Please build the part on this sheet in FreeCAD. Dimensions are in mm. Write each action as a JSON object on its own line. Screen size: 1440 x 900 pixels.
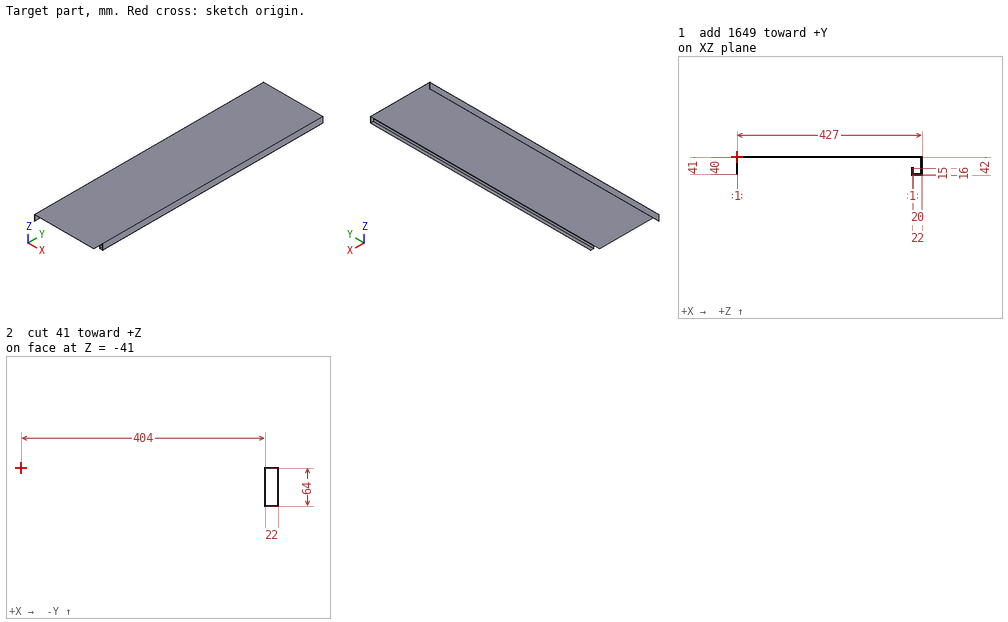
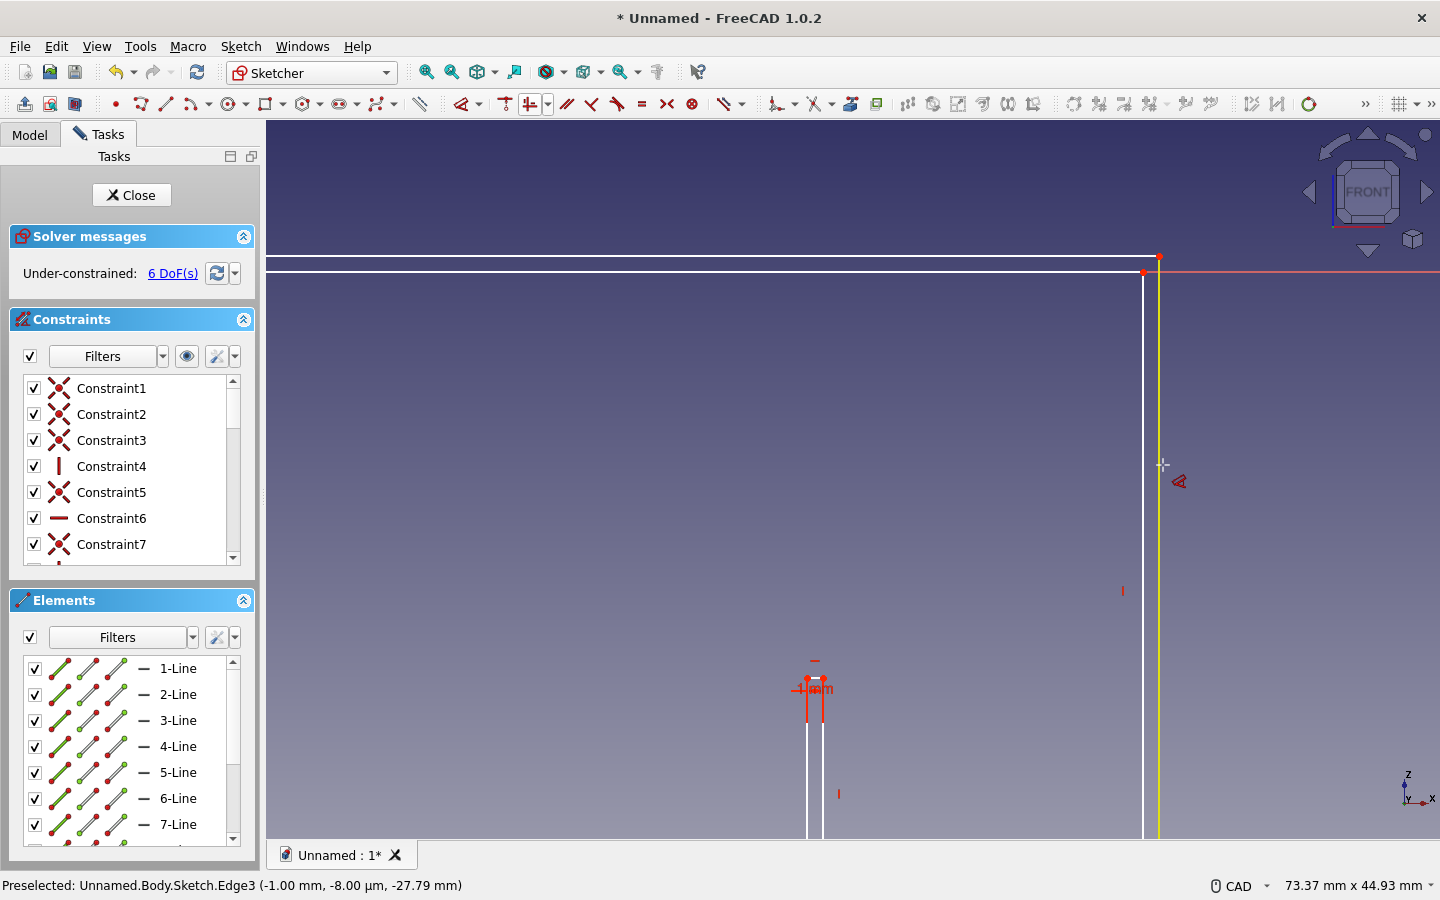
{"action": "left_click", "coordinate": [1159, 461]}
{"action": "left_click", "coordinate": [1193, 534]}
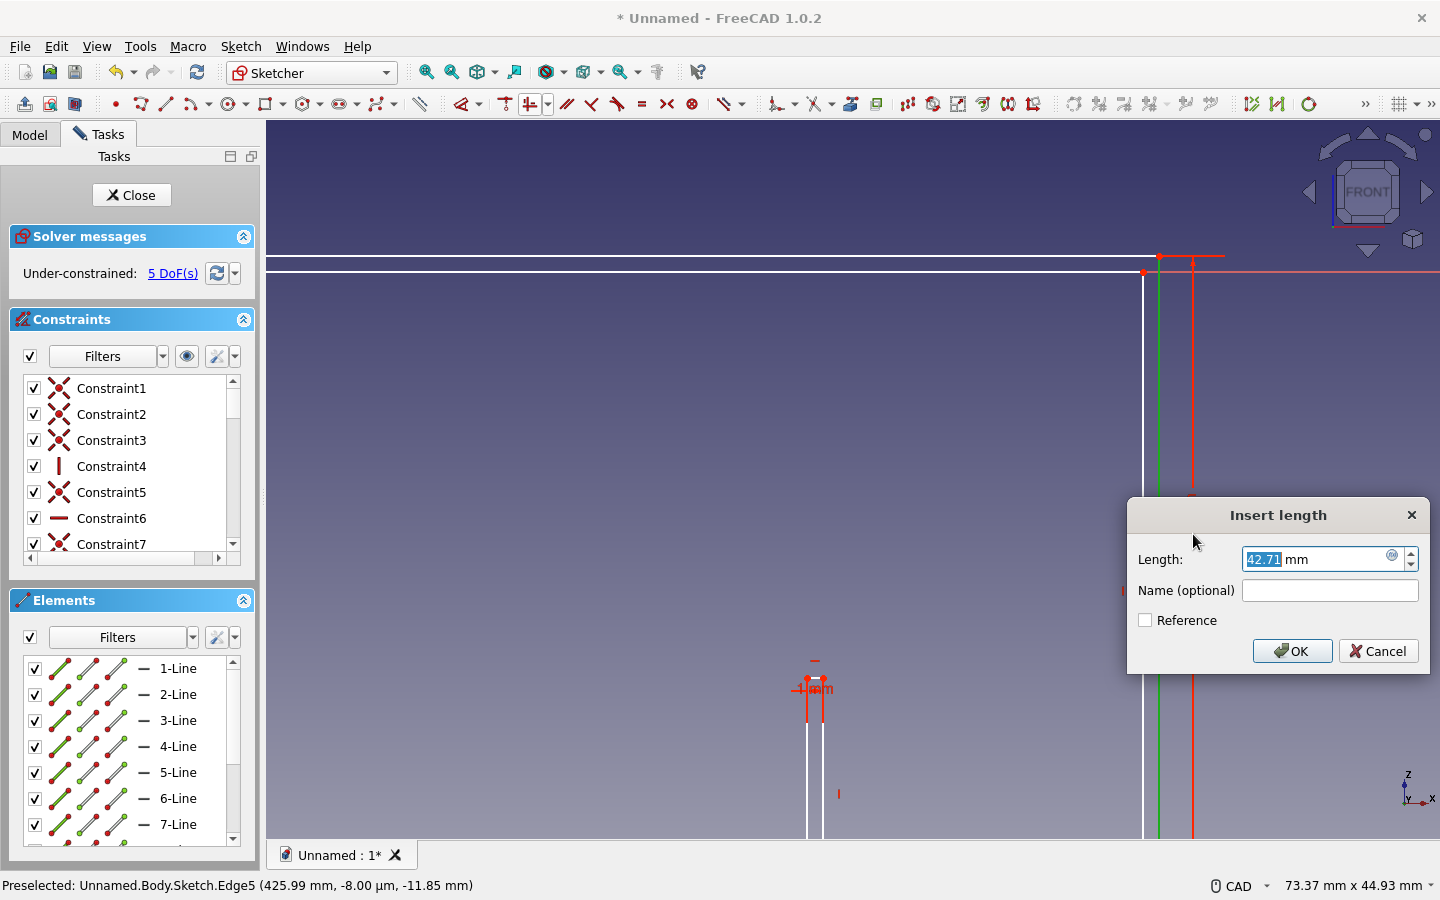
{"action": "type", "text": "42"}
{"action": "key", "text": "Return"}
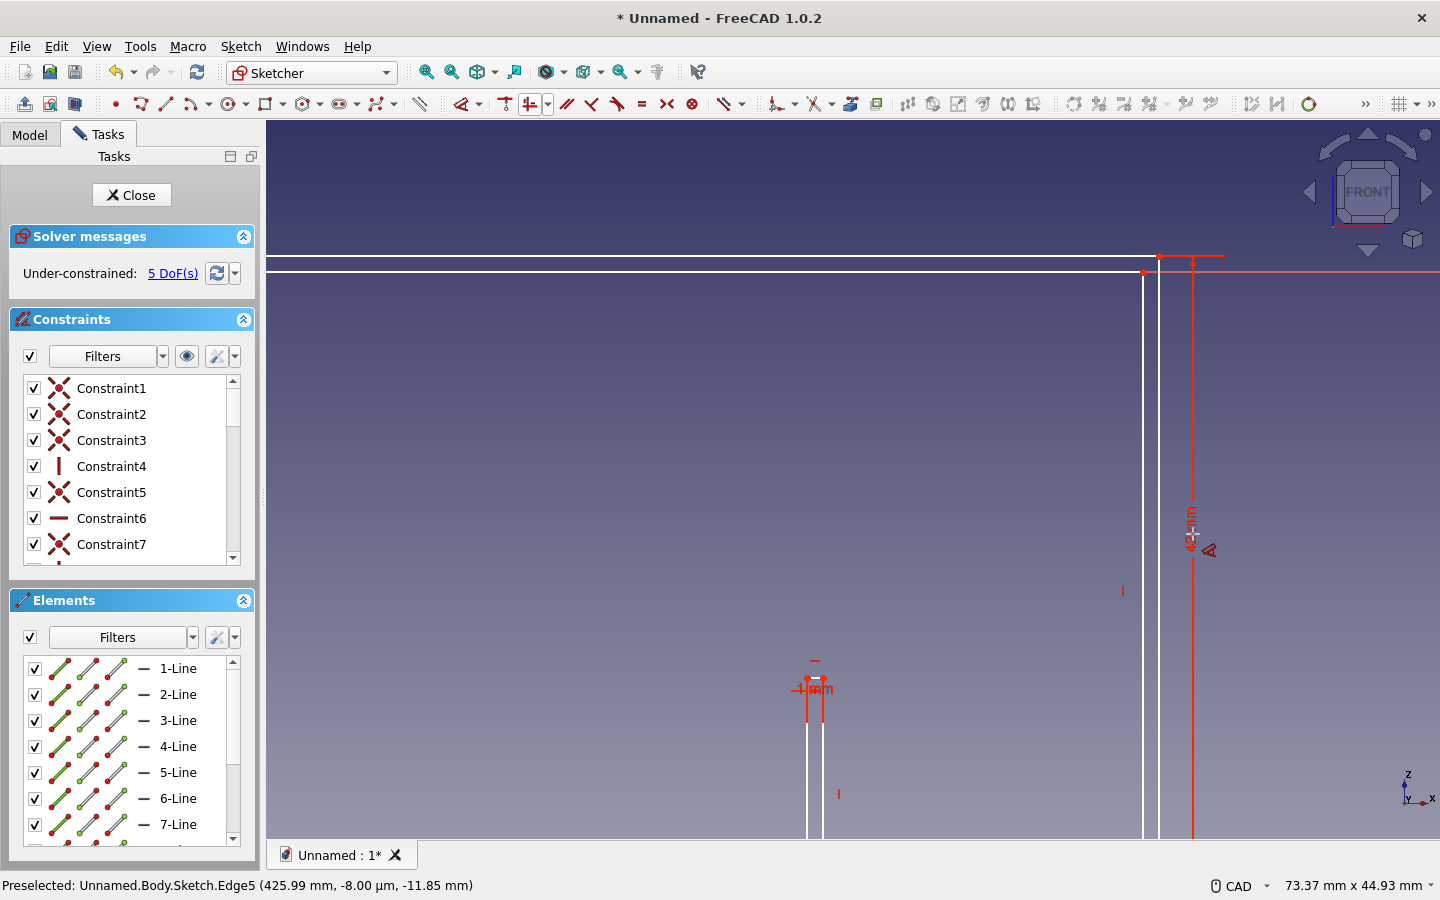
{"action": "scroll", "coordinate": [1164, 465], "scroll_direction": "down", "scroll_amount": 11}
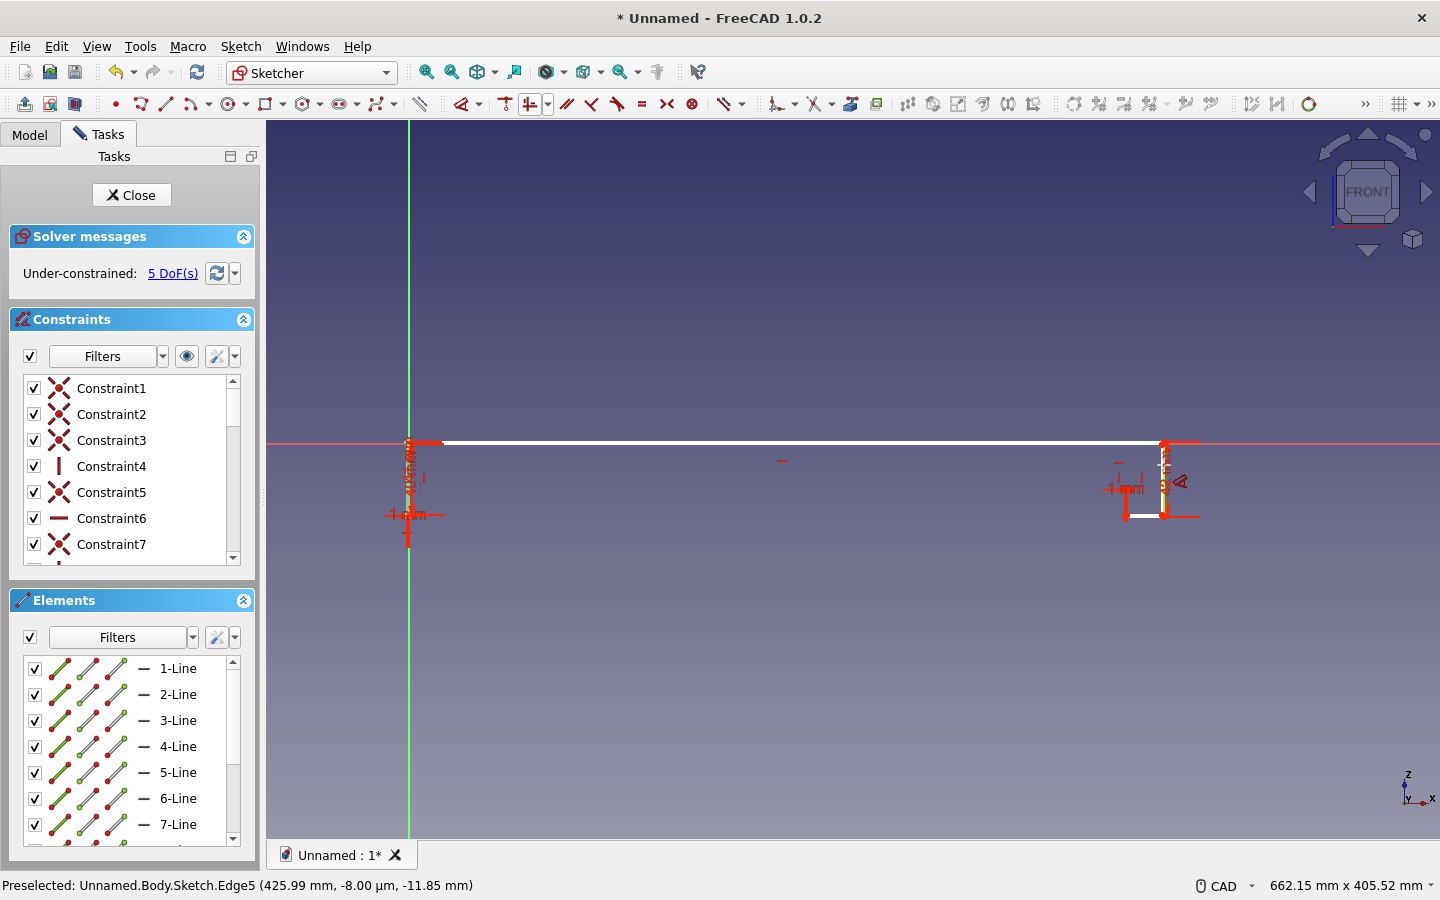
{"action": "scroll", "coordinate": [1152, 517], "scroll_direction": "up", "scroll_amount": 11}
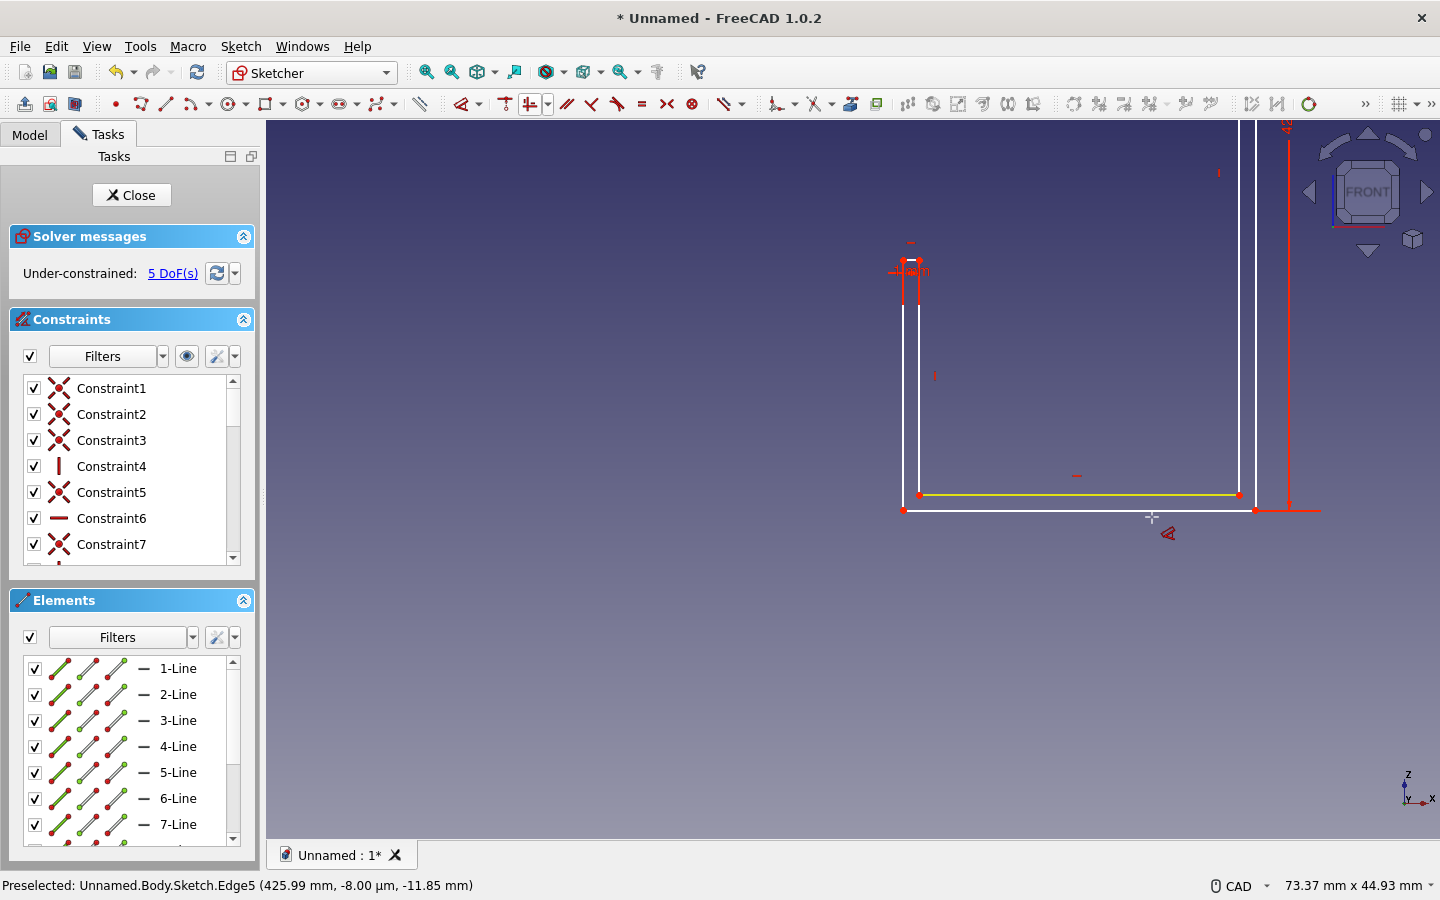
{"action": "left_click", "coordinate": [1150, 511]}
{"action": "left_click", "coordinate": [1079, 545]}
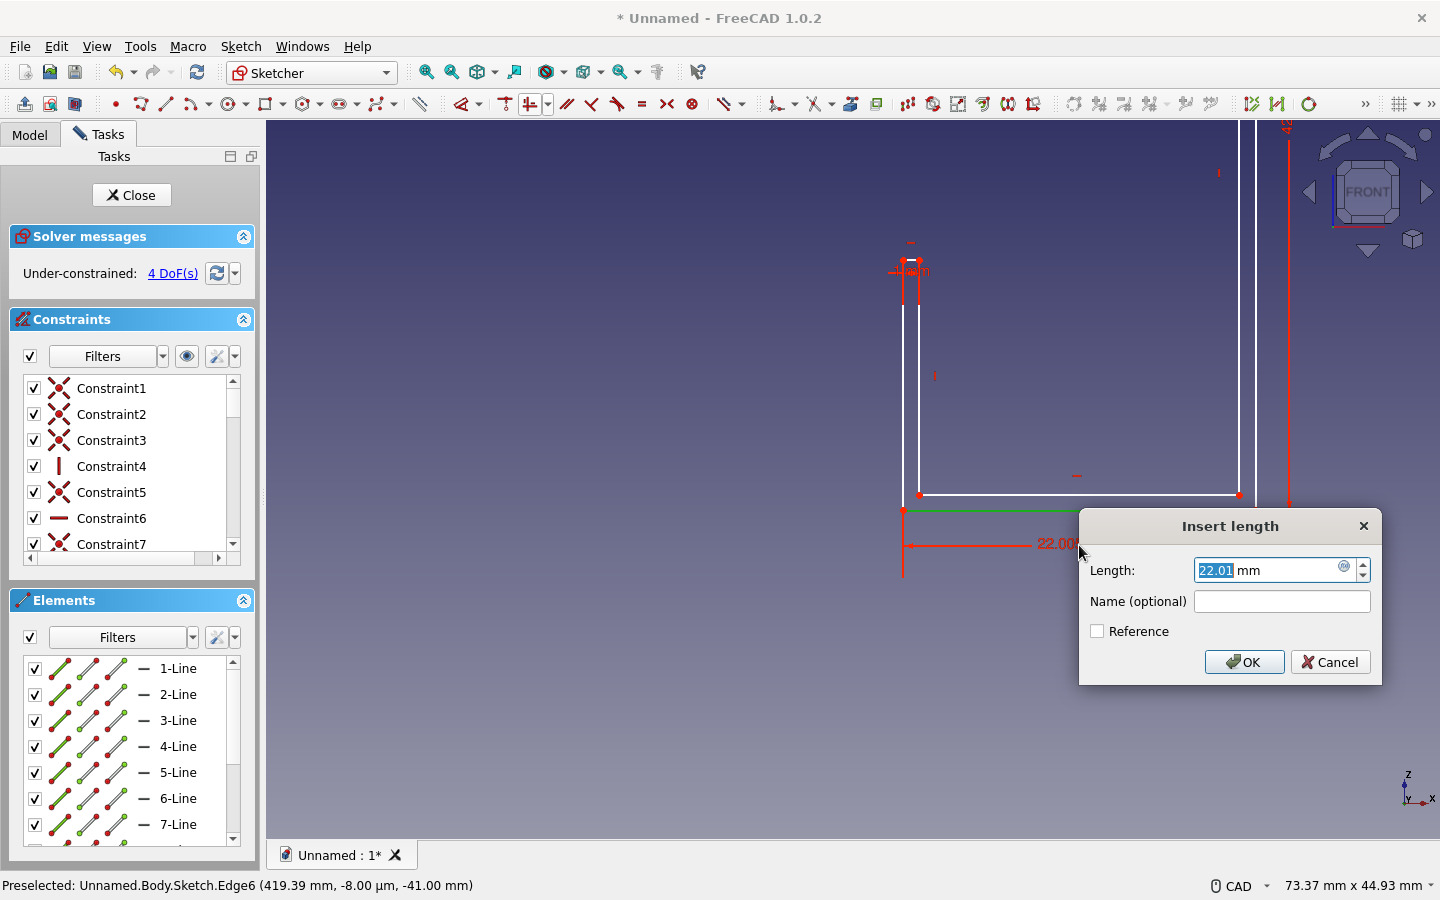
{"action": "type", "text": "22"}
{"action": "key", "text": "Return"}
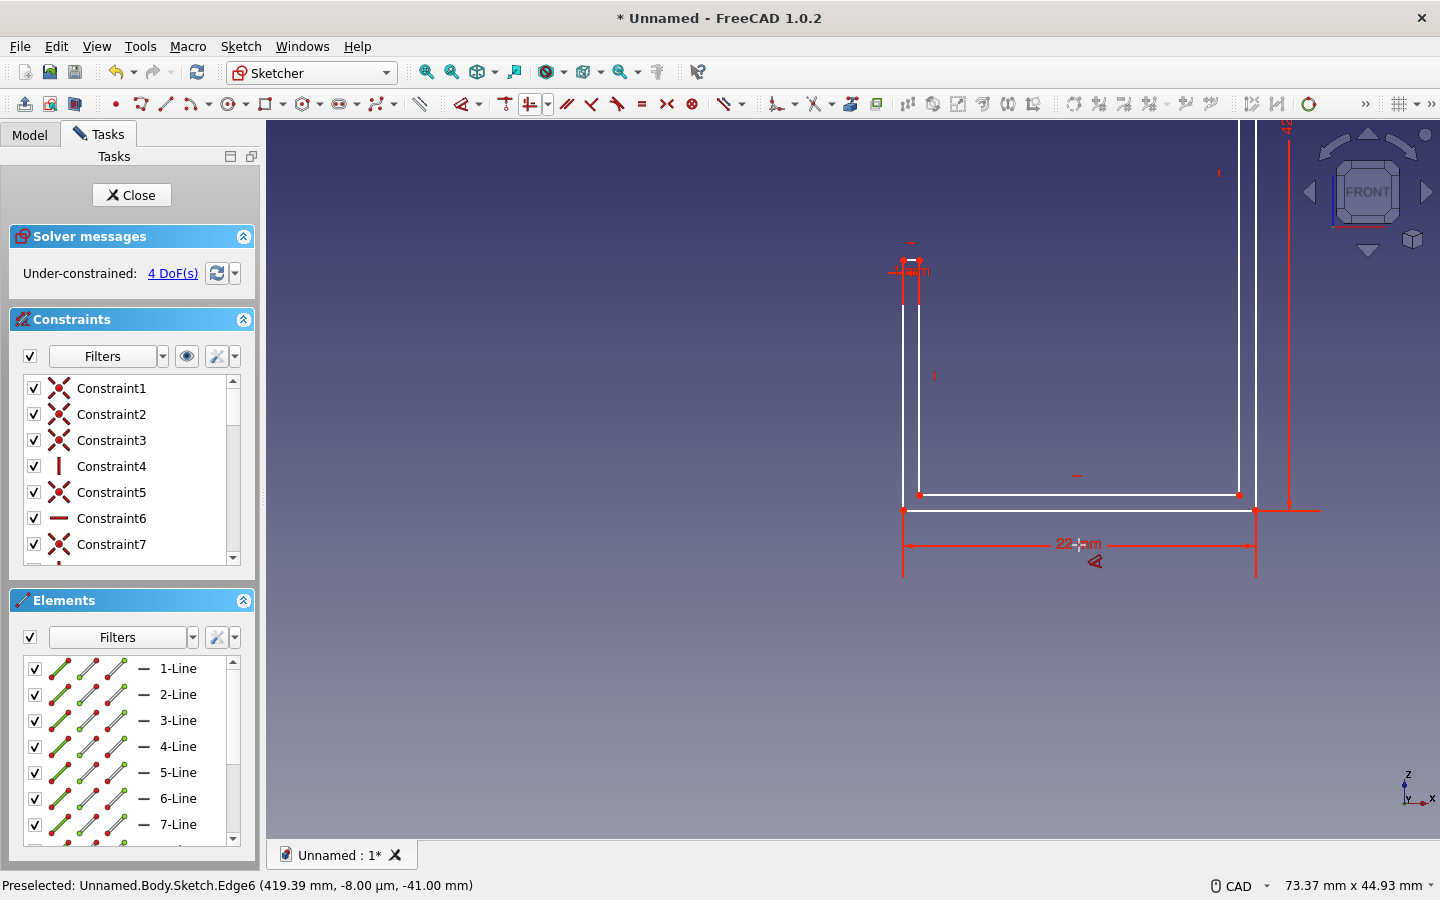
{"action": "left_click", "coordinate": [903, 435]}
{"action": "left_click", "coordinate": [937, 385]}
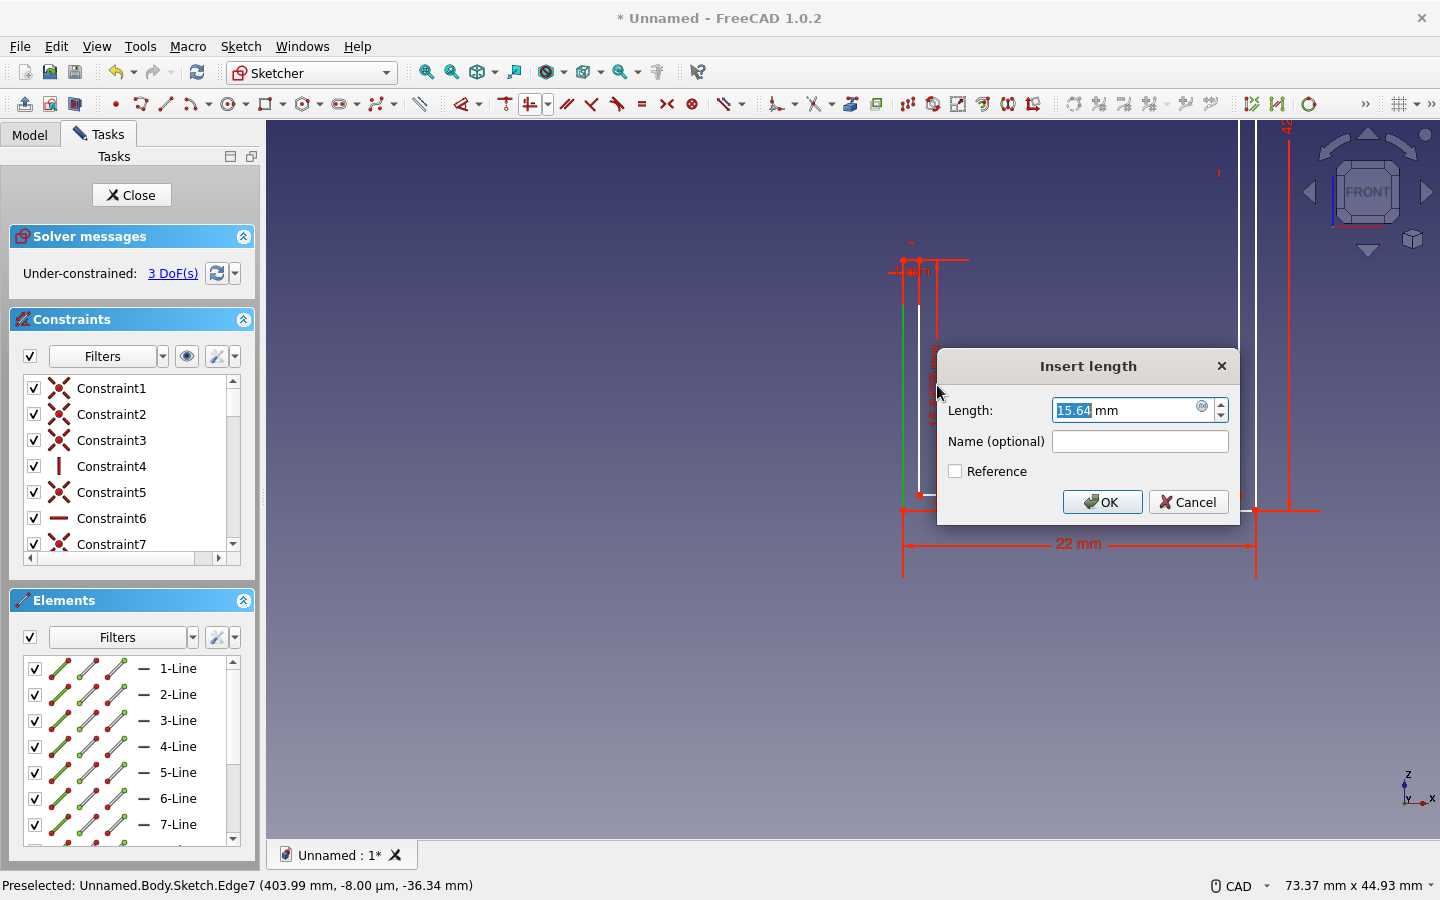
{"action": "type", "text": "16"}
{"action": "key", "text": "Return"}